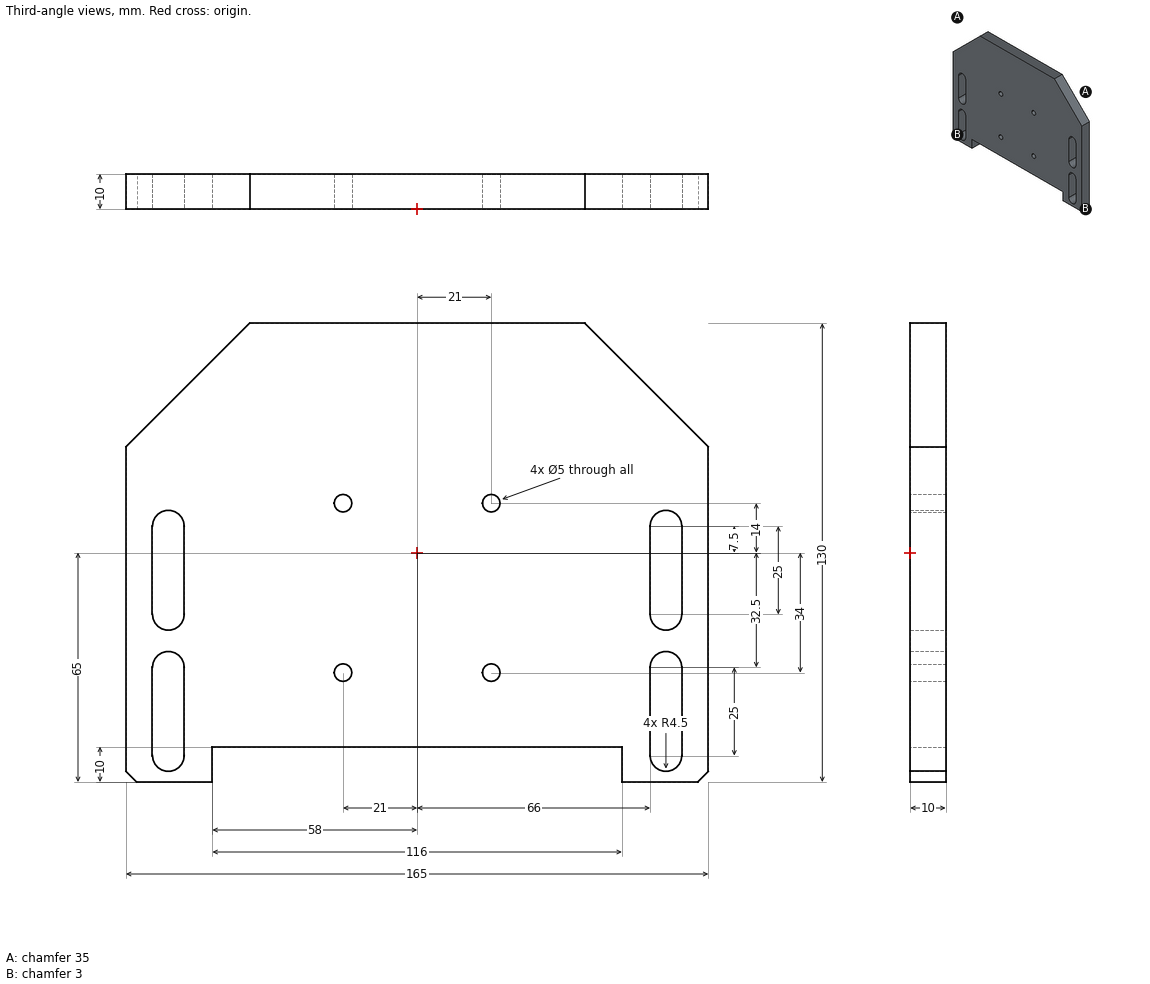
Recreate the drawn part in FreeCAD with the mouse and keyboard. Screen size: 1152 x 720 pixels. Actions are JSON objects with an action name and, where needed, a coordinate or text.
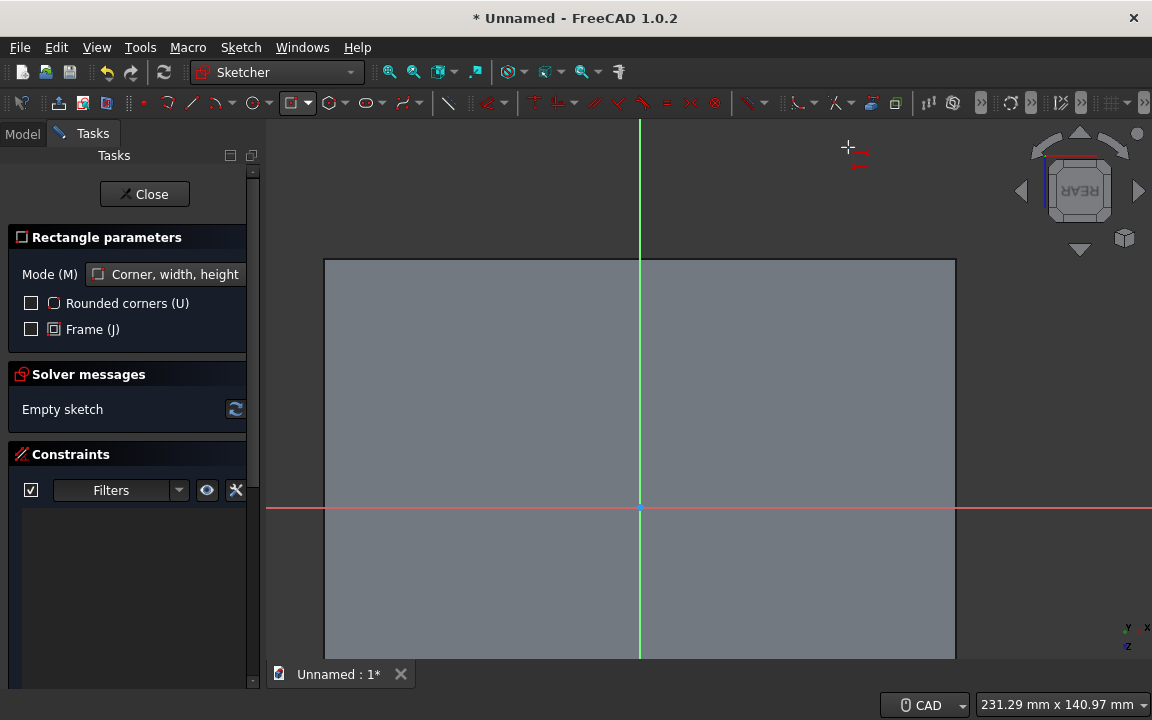
{"action": "left_click", "coordinate": [418, 259]}
{"action": "left_click", "coordinate": [862, 297]}
{"action": "key", "text": "Escape"}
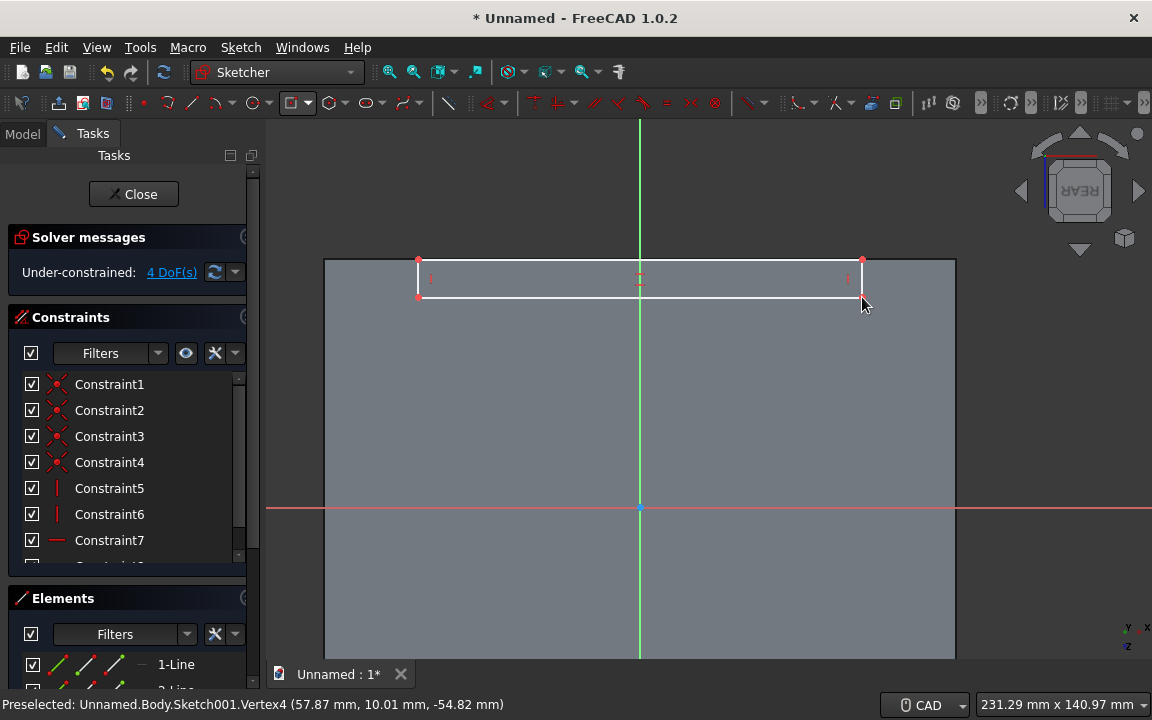
{"action": "left_click", "coordinate": [488, 104]}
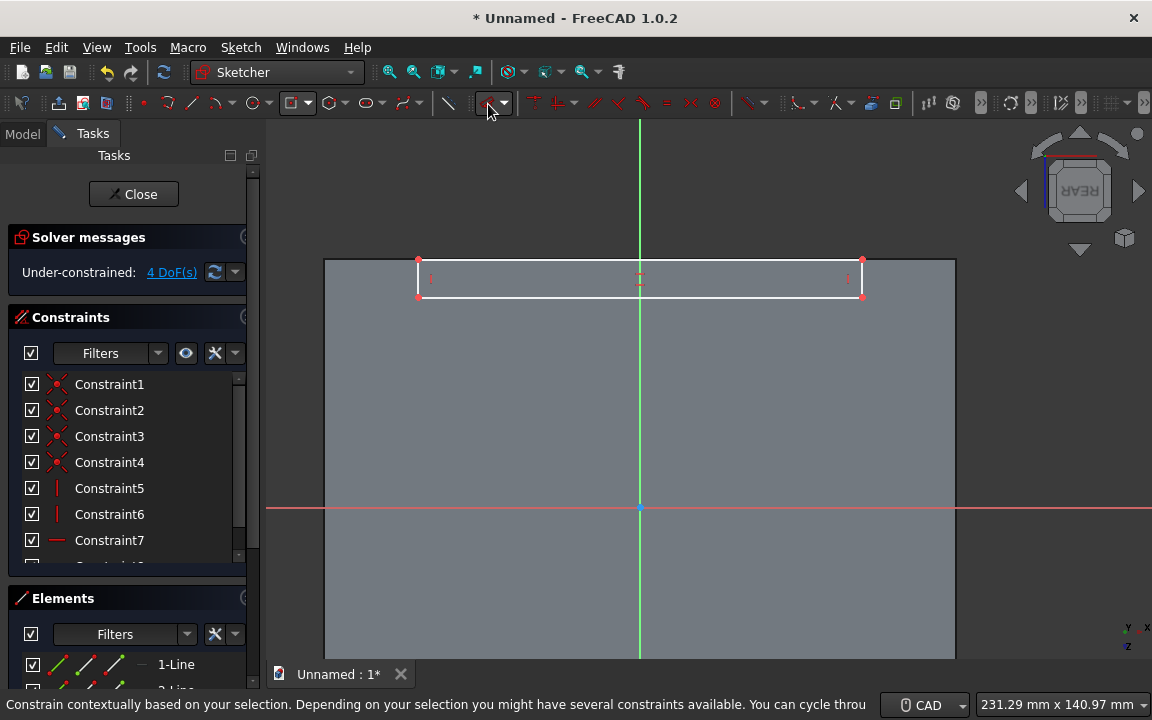
{"action": "left_click", "coordinate": [418, 271]}
{"action": "left_click", "coordinate": [384, 279]}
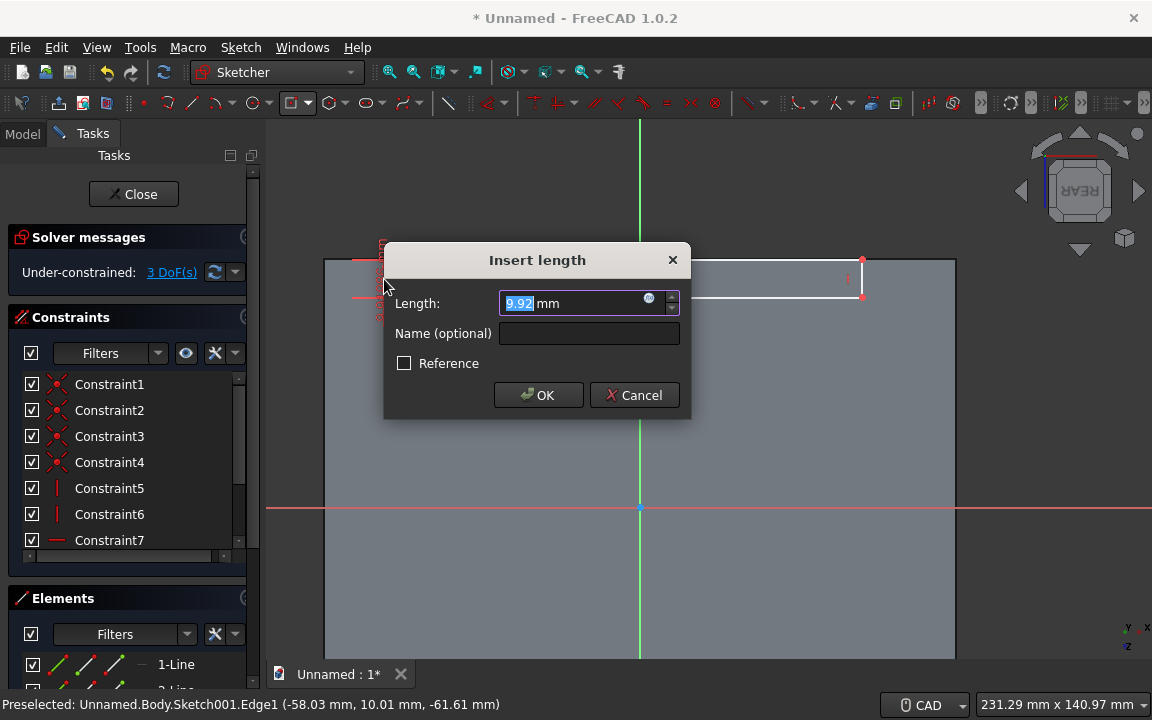
{"action": "type", "text": "10"}
{"action": "key", "text": "Return"}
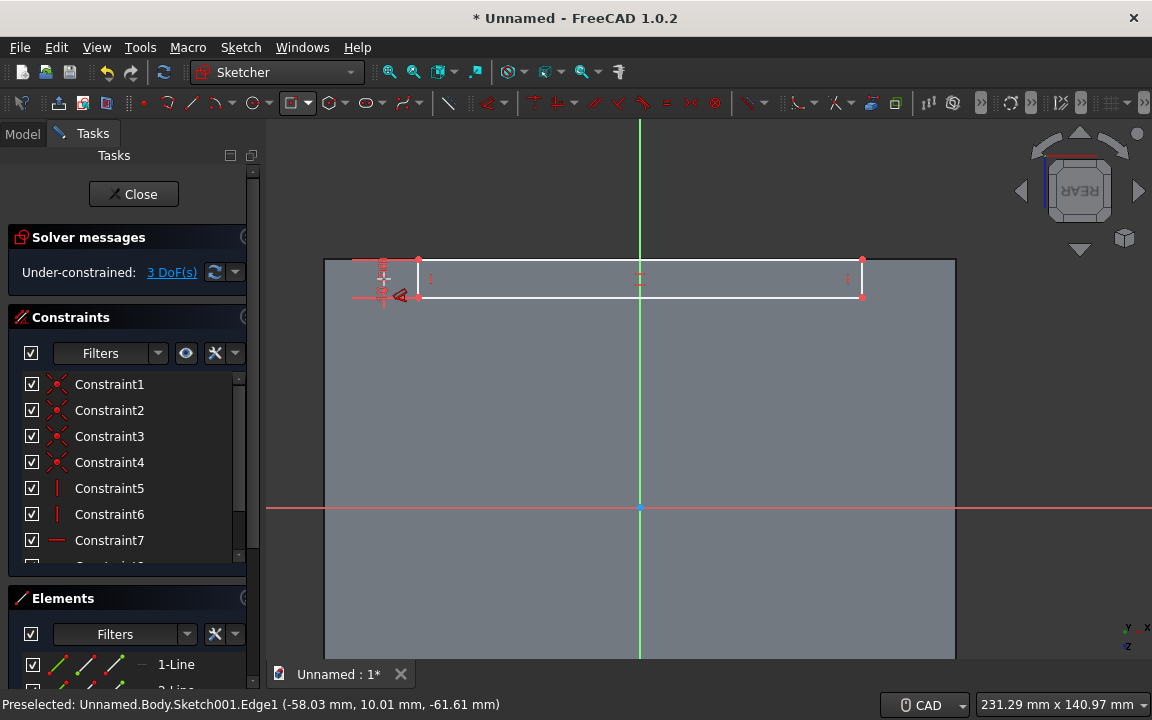
{"action": "left_click", "coordinate": [551, 298]}
{"action": "left_click", "coordinate": [538, 332]}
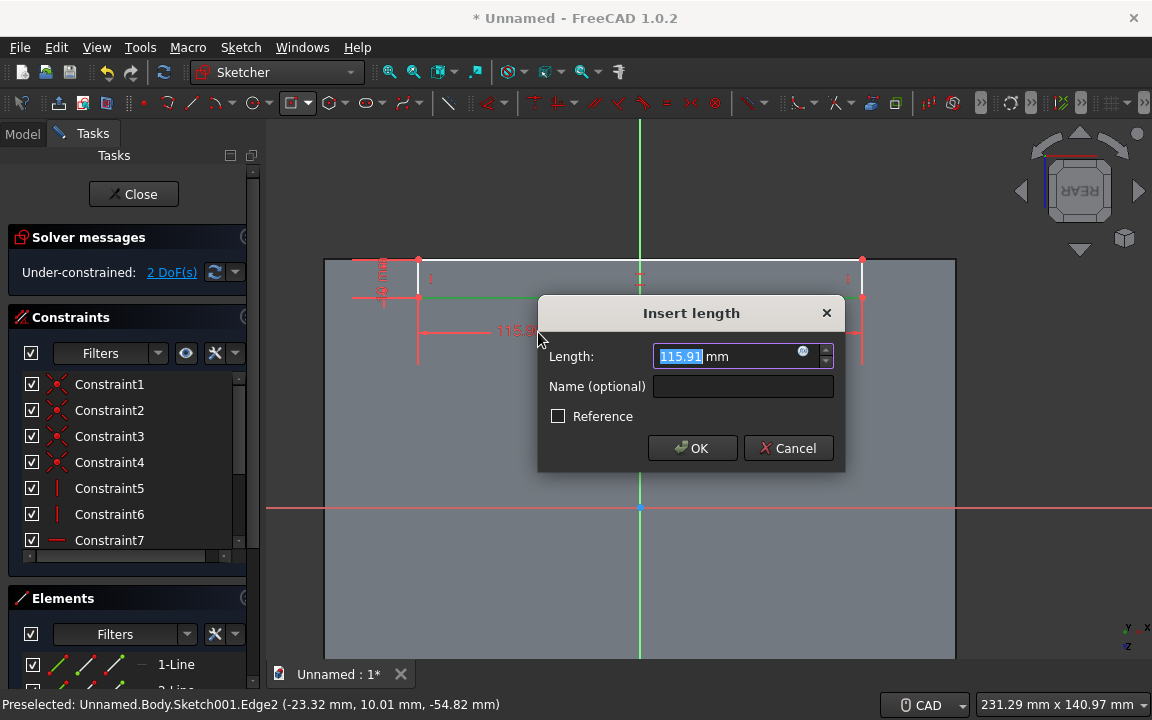
{"action": "type", "text": "116"}
{"action": "key", "text": "Return"}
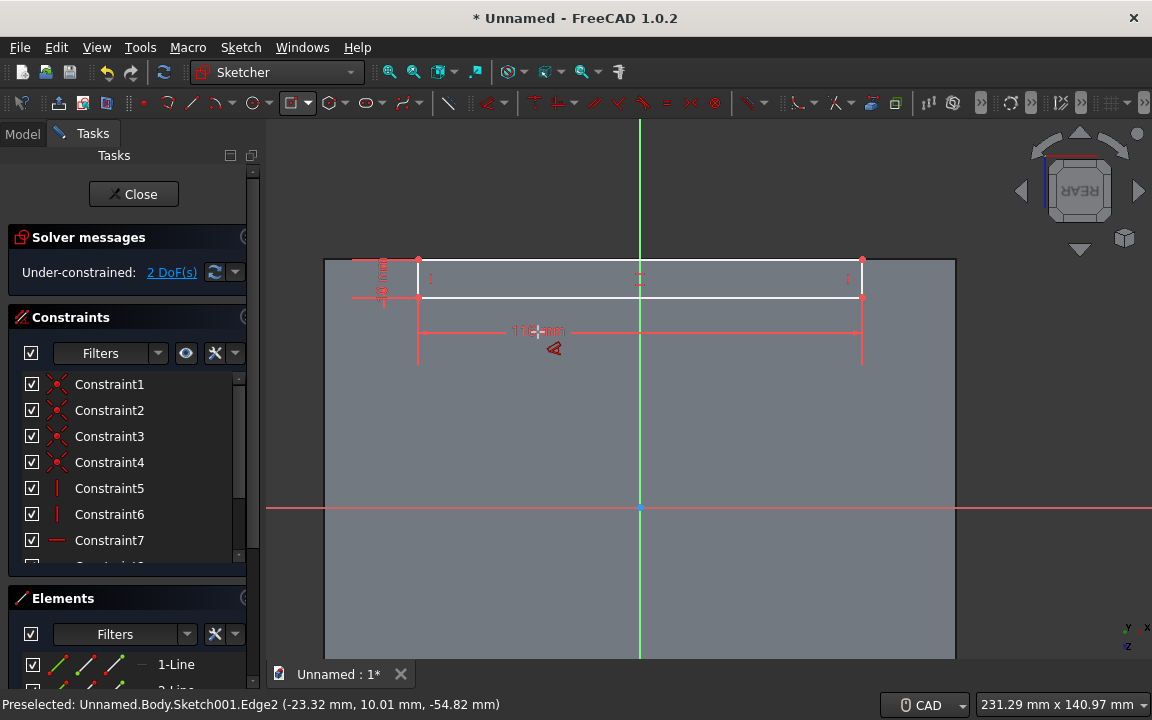
{"action": "left_click", "coordinate": [418, 260]}
{"action": "left_click", "coordinate": [529, 542]}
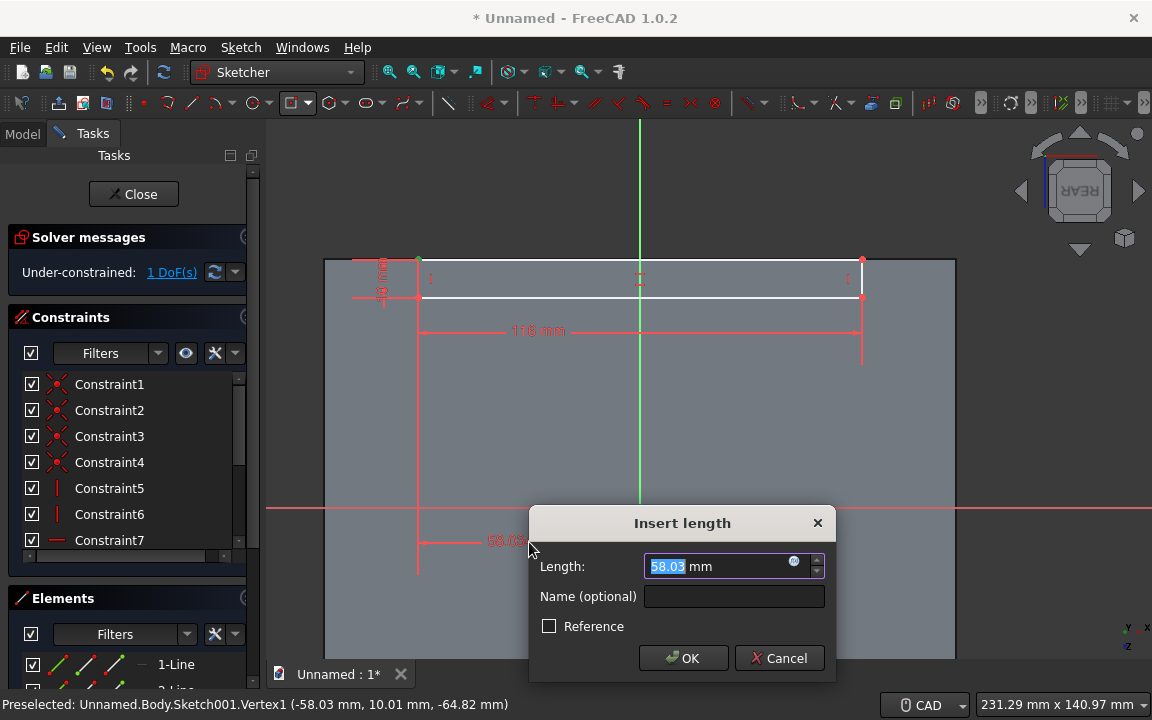
{"action": "type", "text": "58"}
{"action": "key", "text": "Return"}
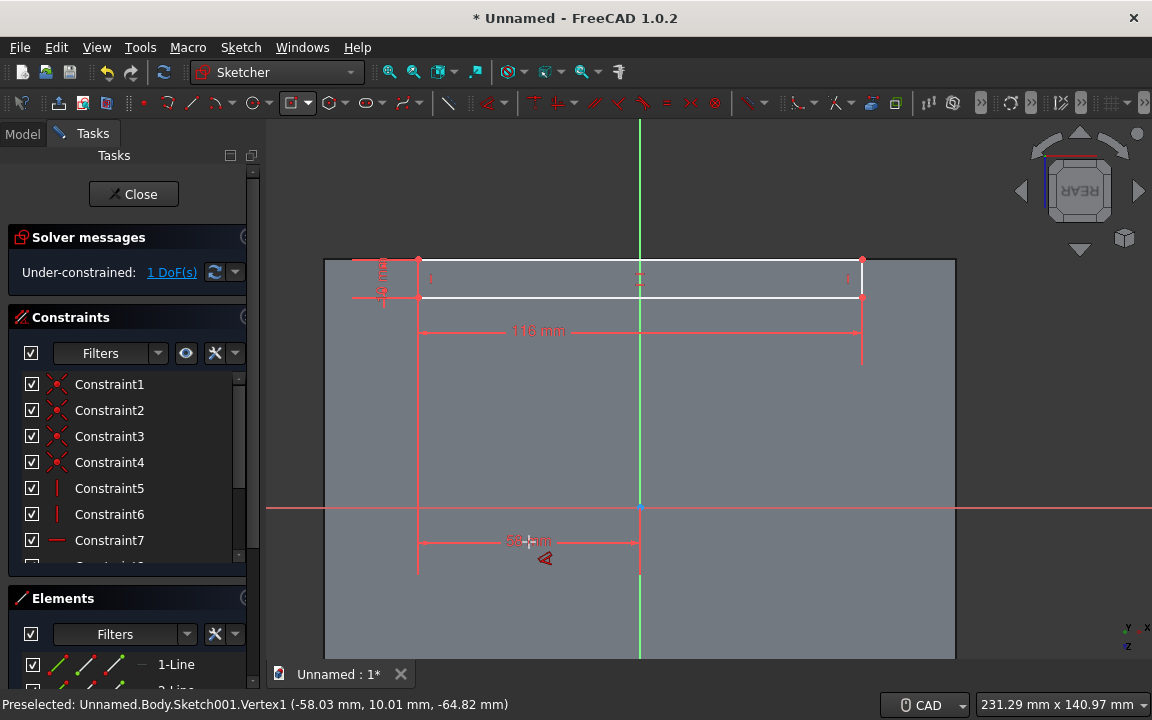
{"action": "left_click", "coordinate": [418, 260]}
{"action": "left_click", "coordinate": [384, 384]}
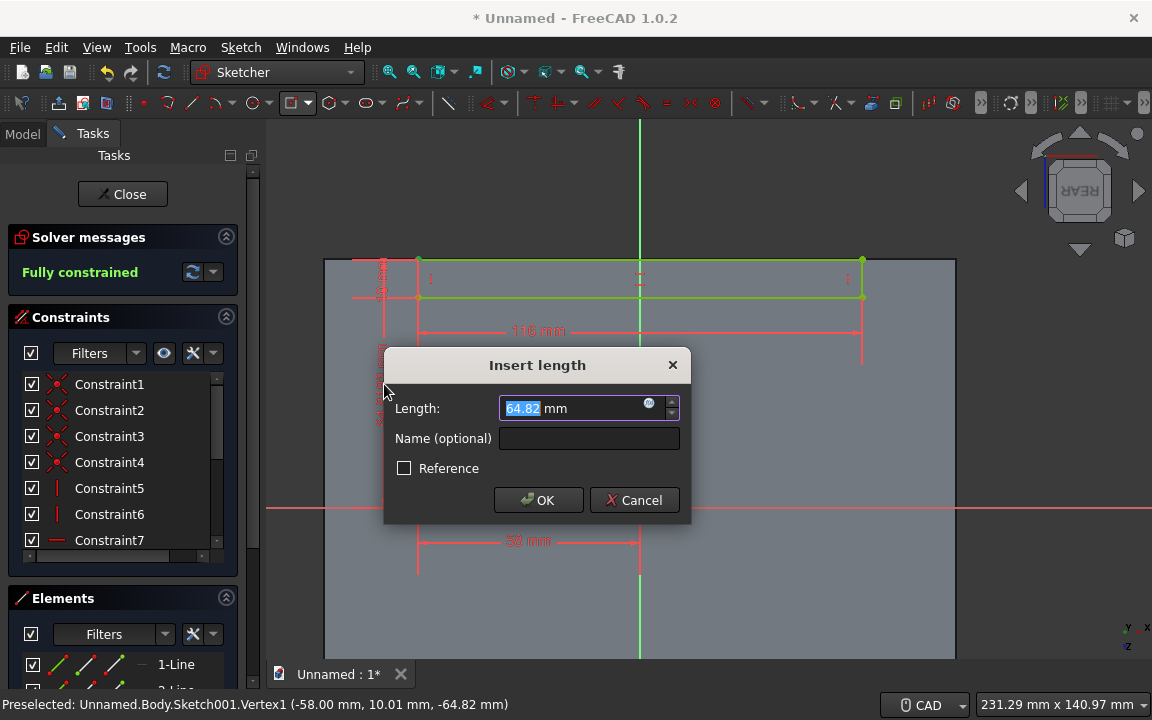
{"action": "type", "text": "65"}
{"action": "key", "text": "Return"}
{"action": "key", "text": "Escape"}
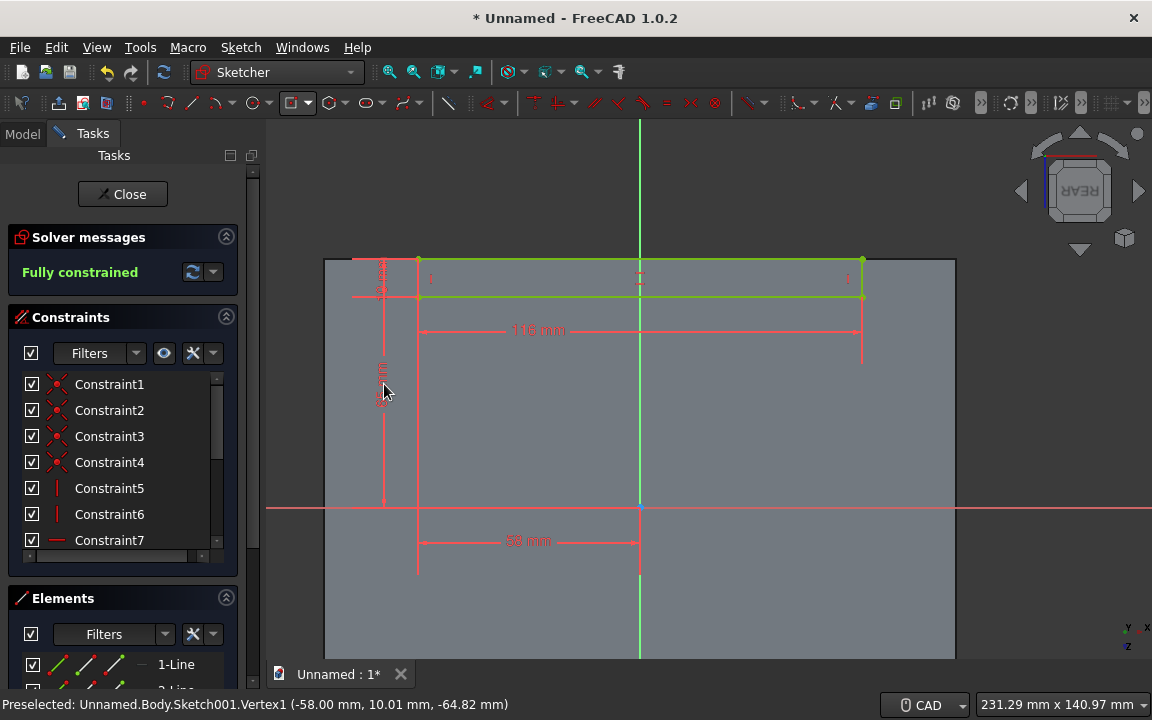
{"action": "left_click", "coordinate": [123, 194]}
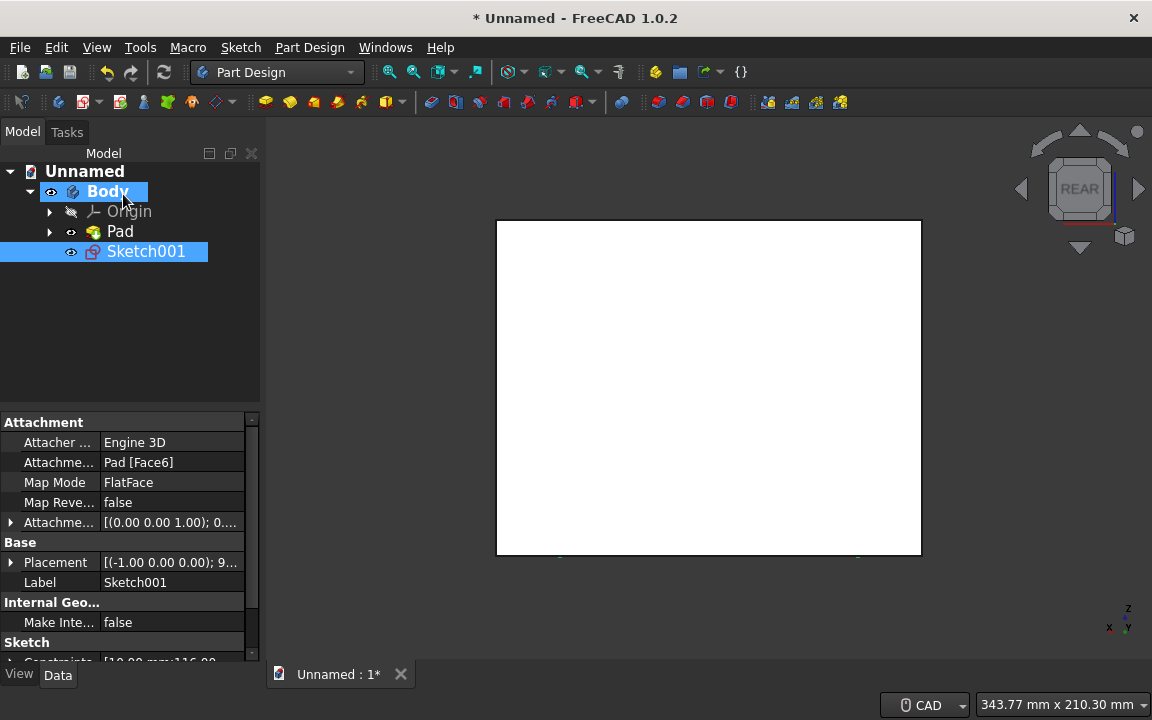
{"action": "left_click", "coordinate": [432, 102]}